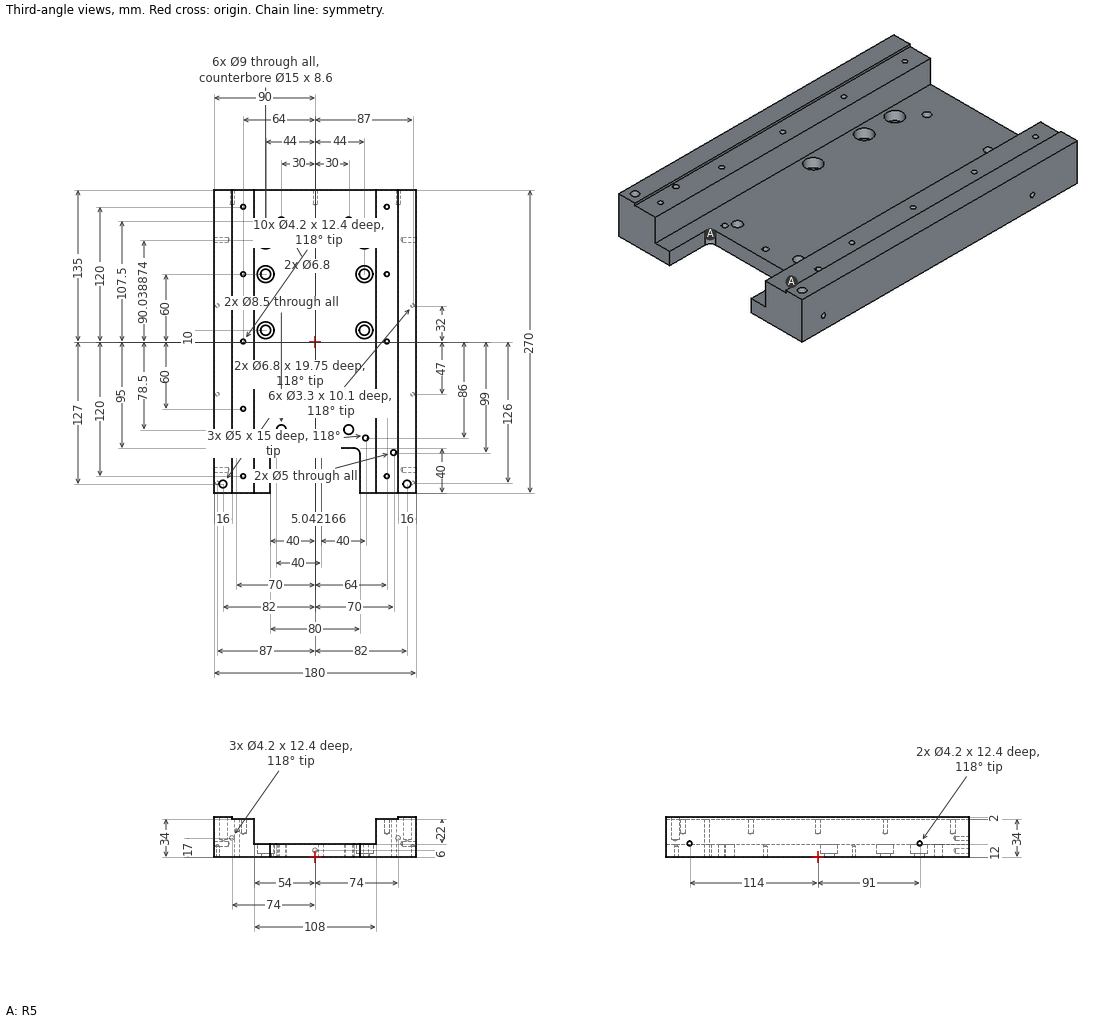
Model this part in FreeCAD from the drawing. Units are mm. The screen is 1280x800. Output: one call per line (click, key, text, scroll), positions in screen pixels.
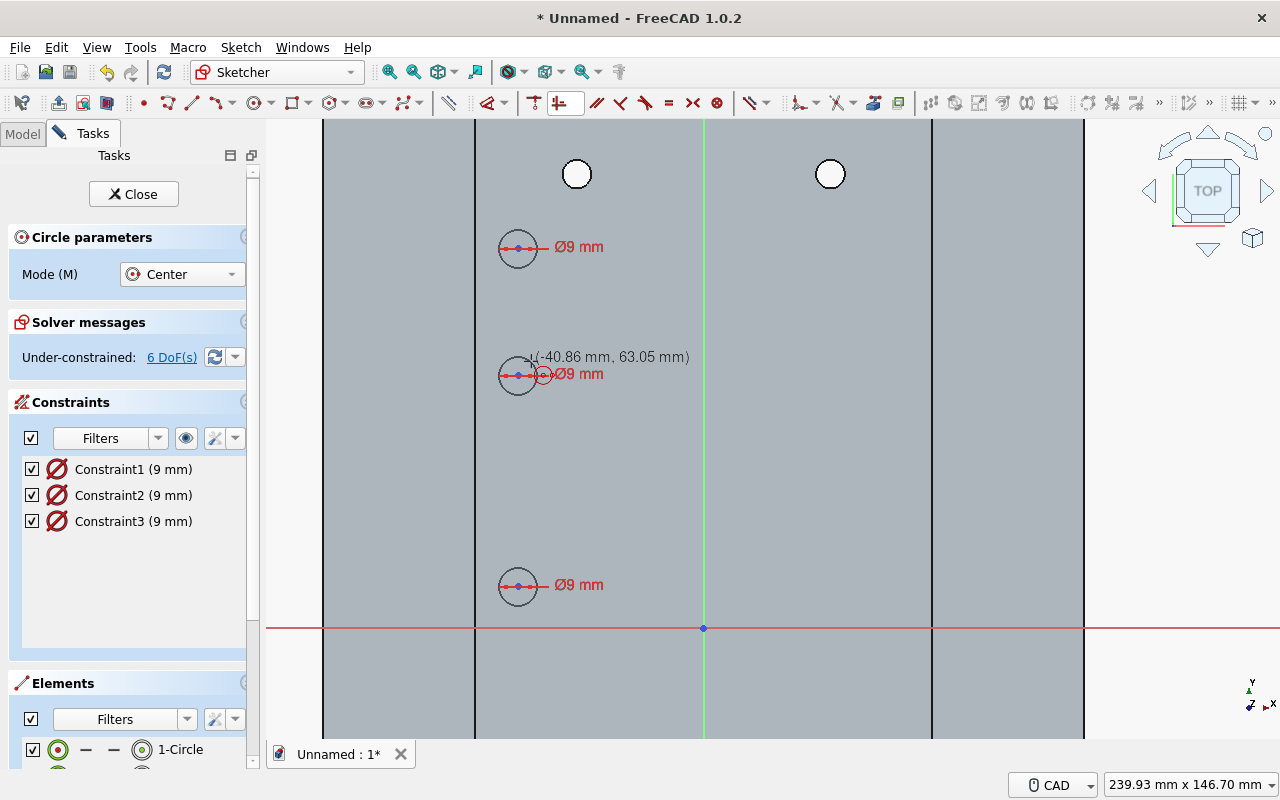
click(890, 375)
move(903, 361)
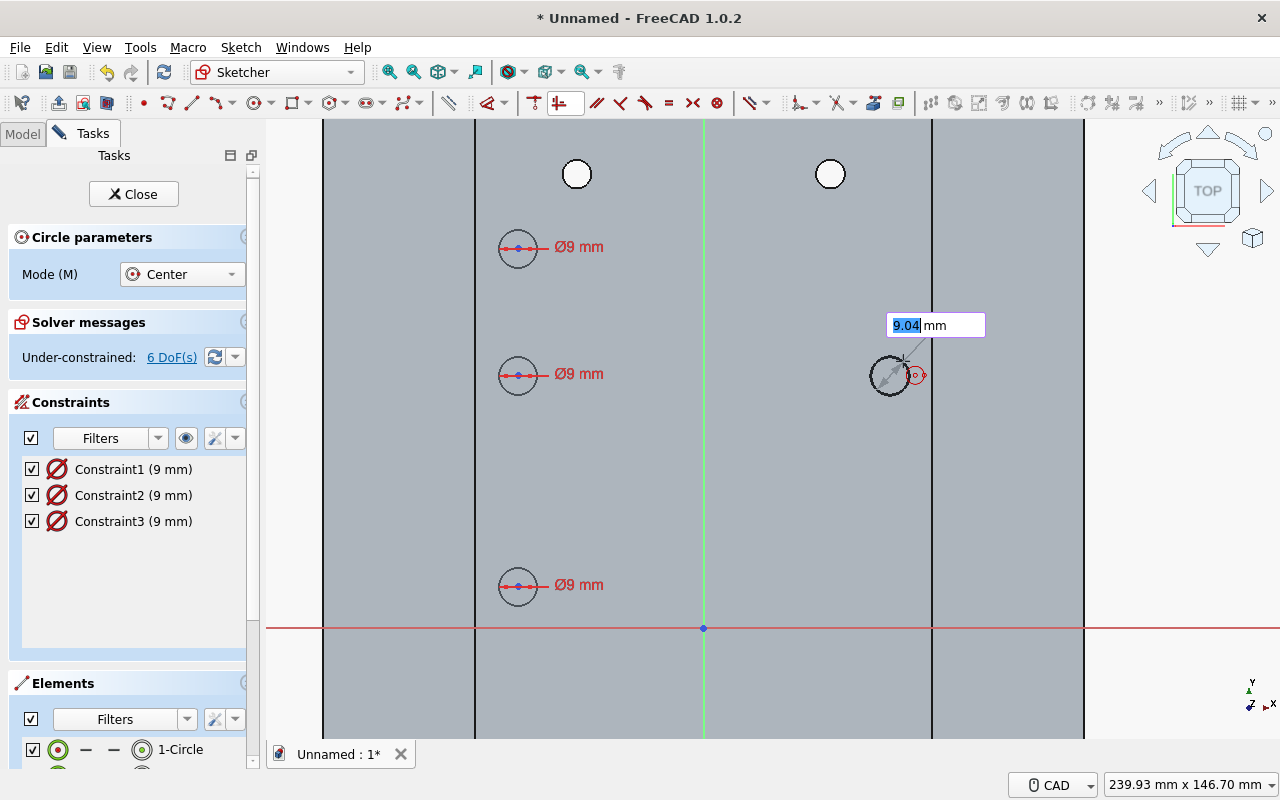
text(9)
key(Return)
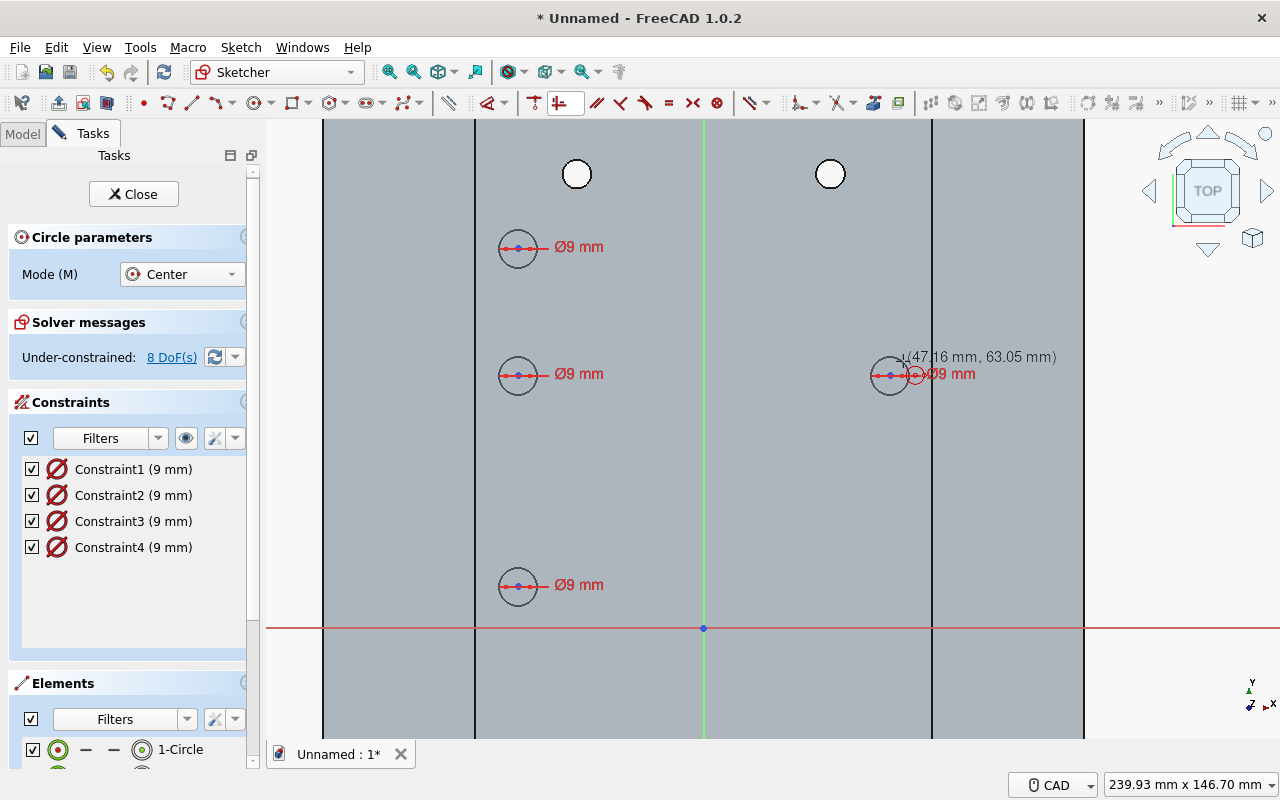
click(890, 586)
move(903, 573)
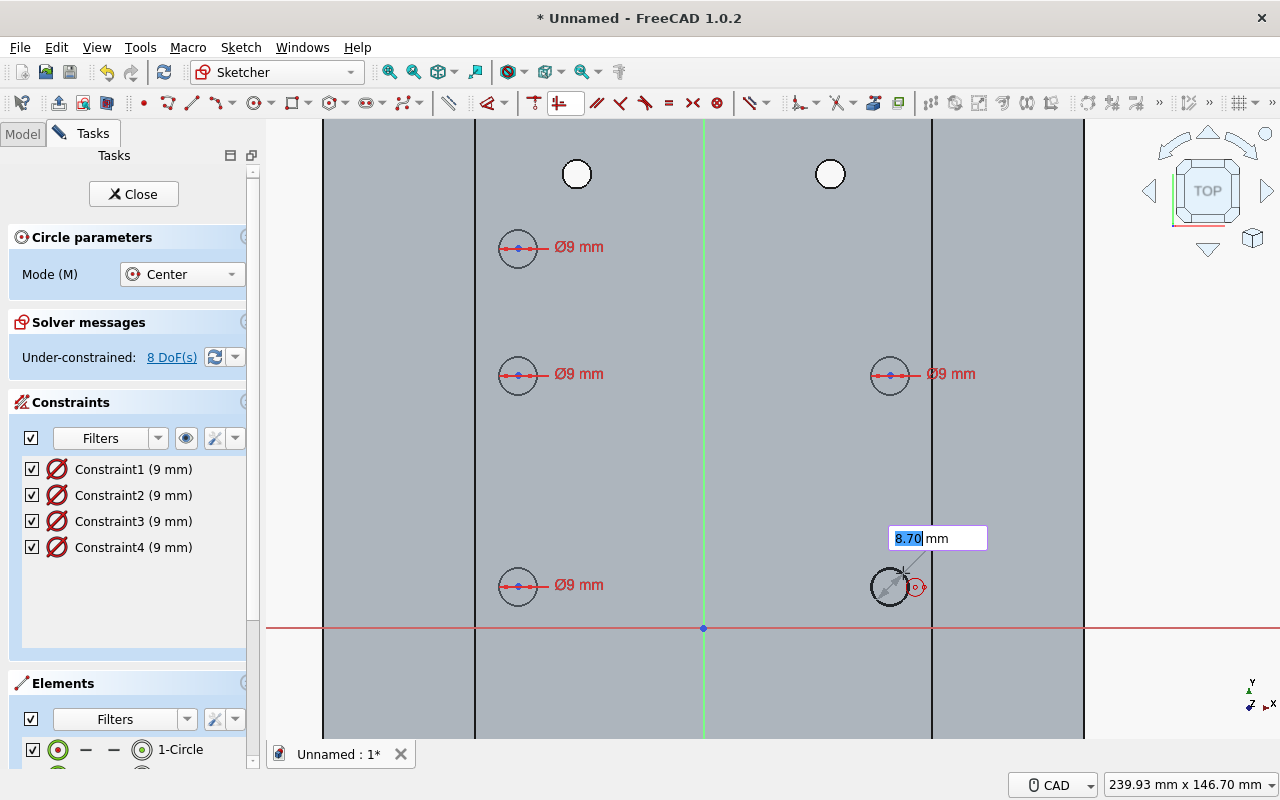
text(9)
key(Return)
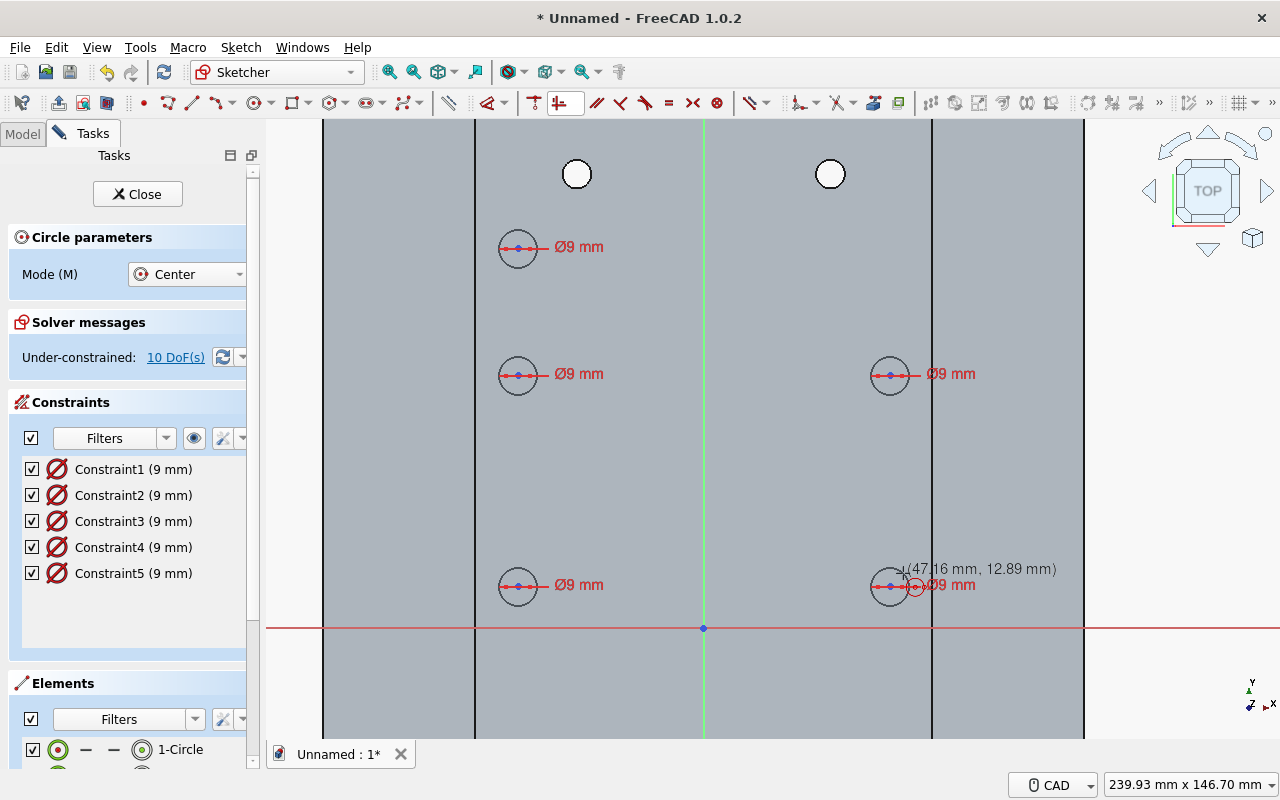
click(890, 248)
move(903, 234)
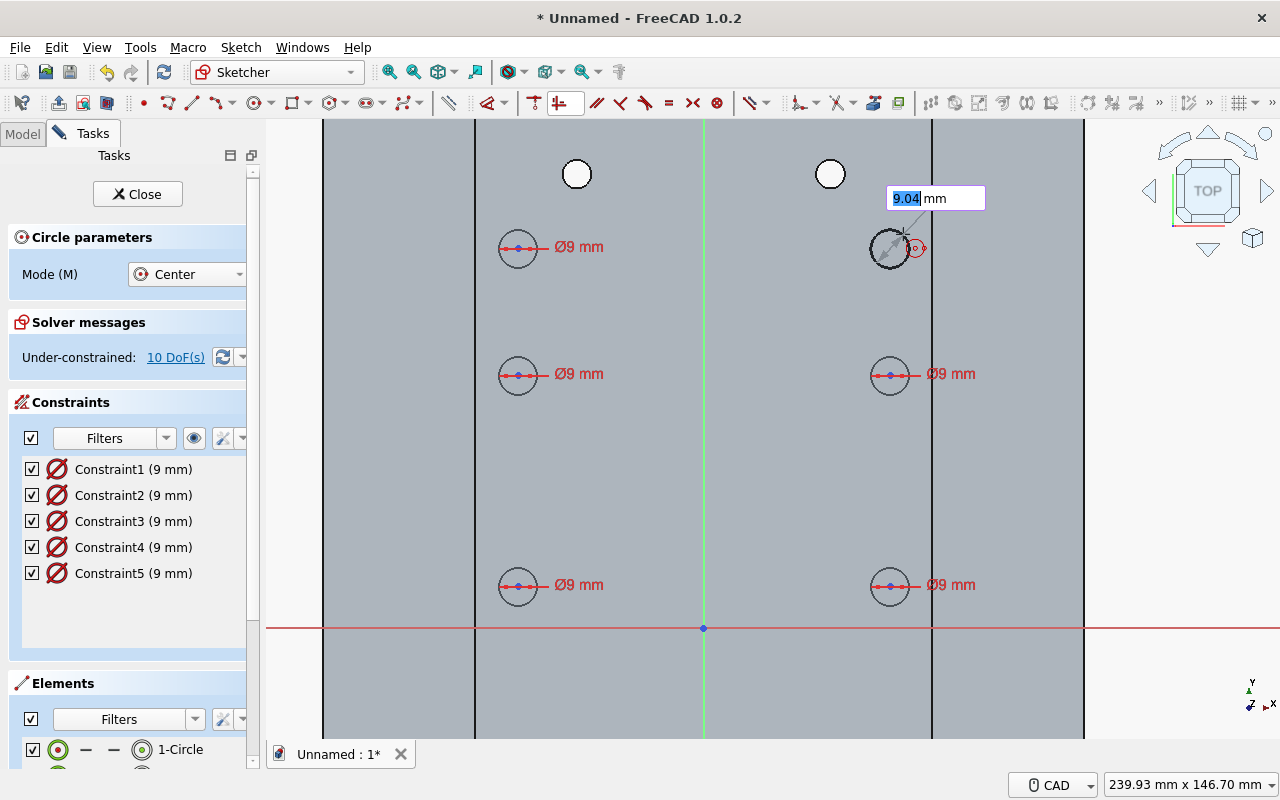
text(9)
key(Return)
key(Escape)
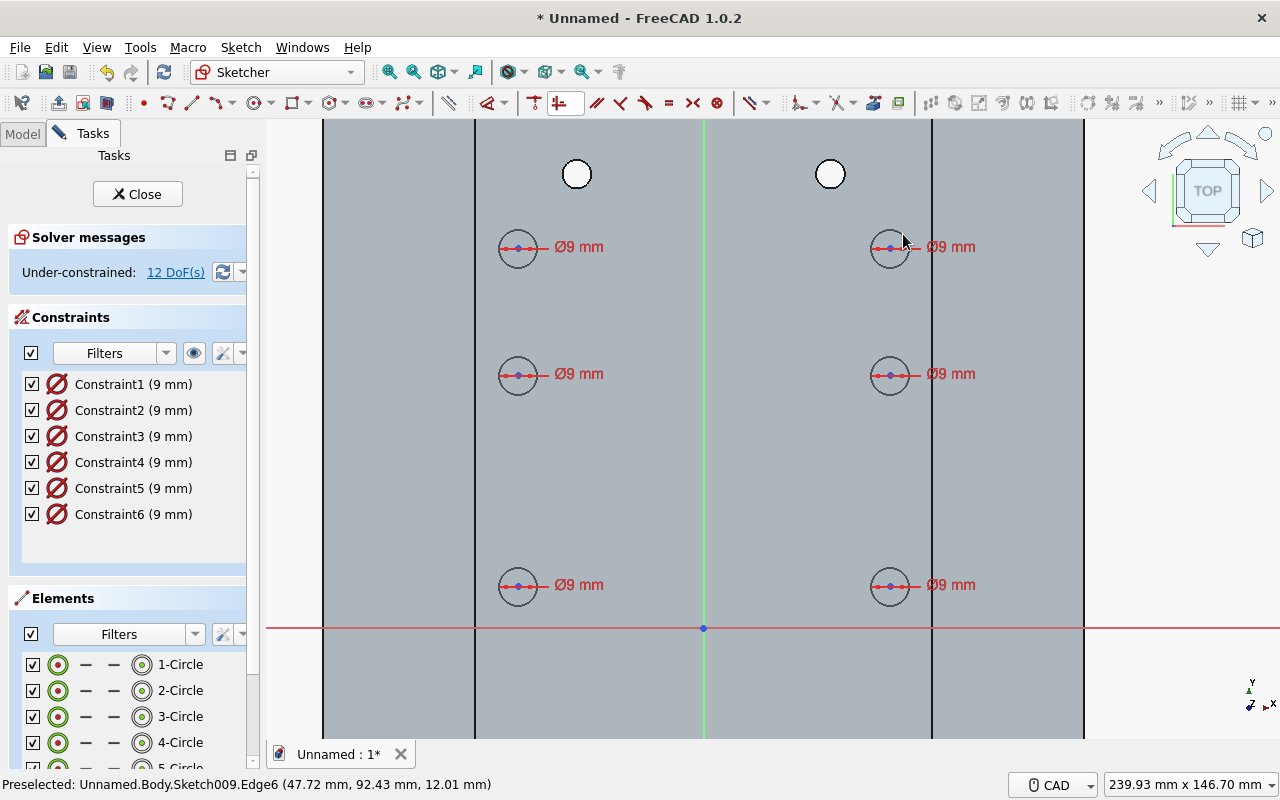
click(518, 249)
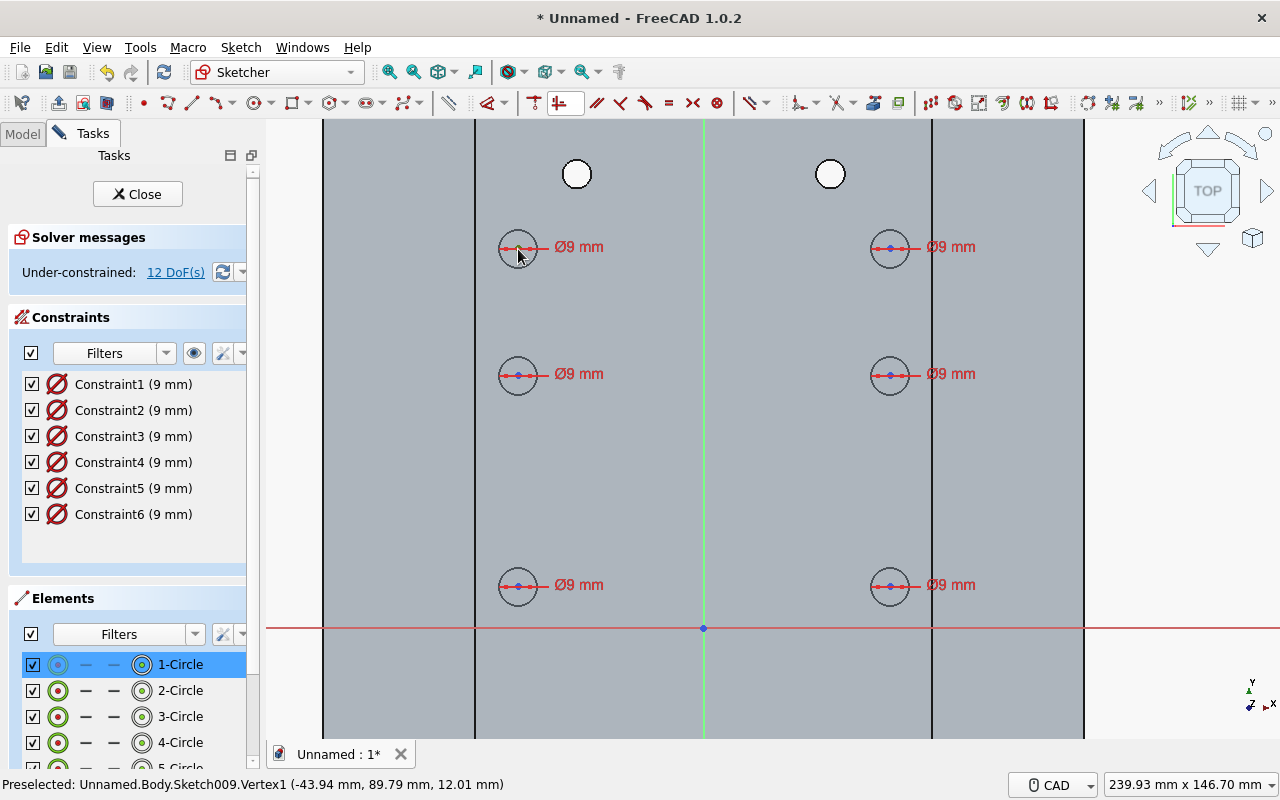
click(518, 587)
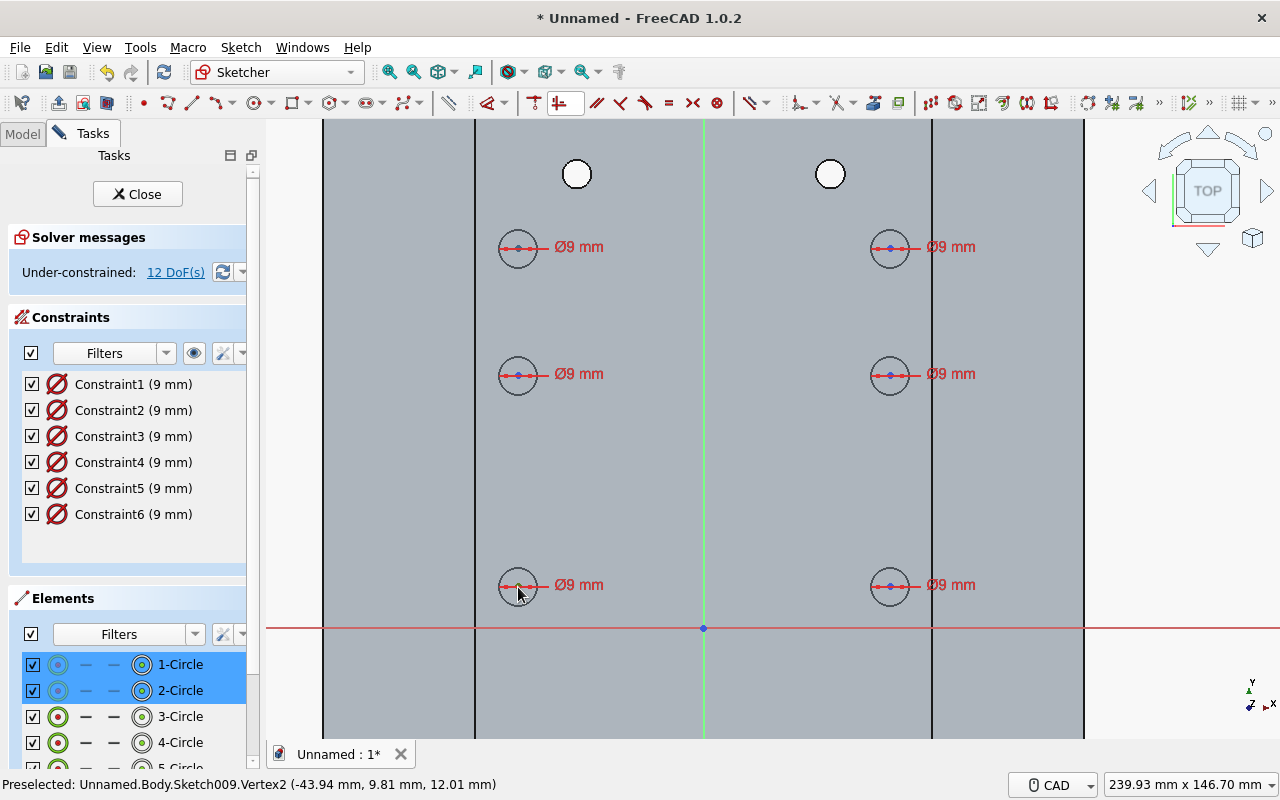
key(v)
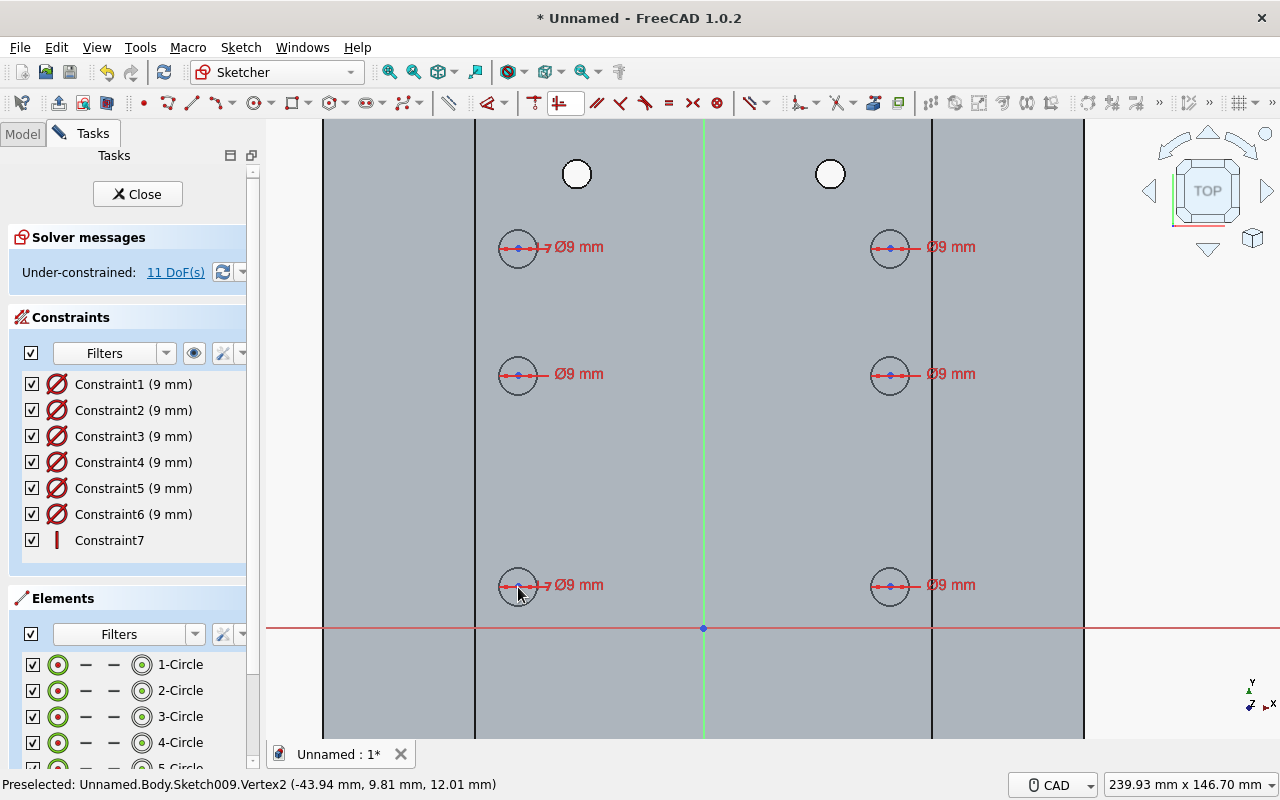
click(518, 249)